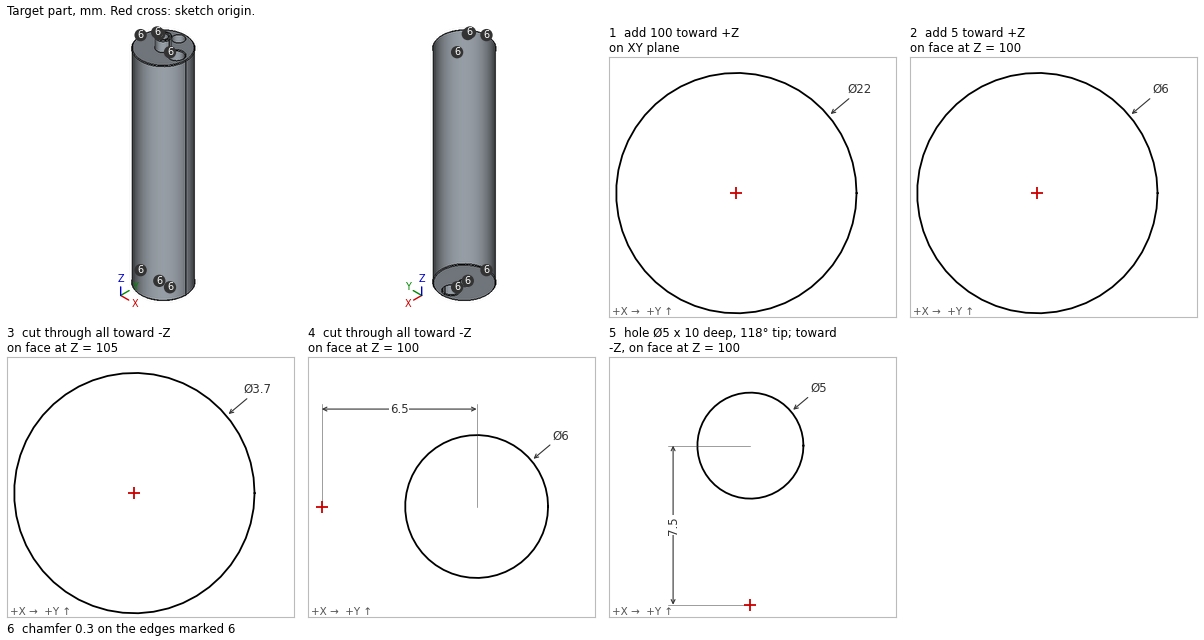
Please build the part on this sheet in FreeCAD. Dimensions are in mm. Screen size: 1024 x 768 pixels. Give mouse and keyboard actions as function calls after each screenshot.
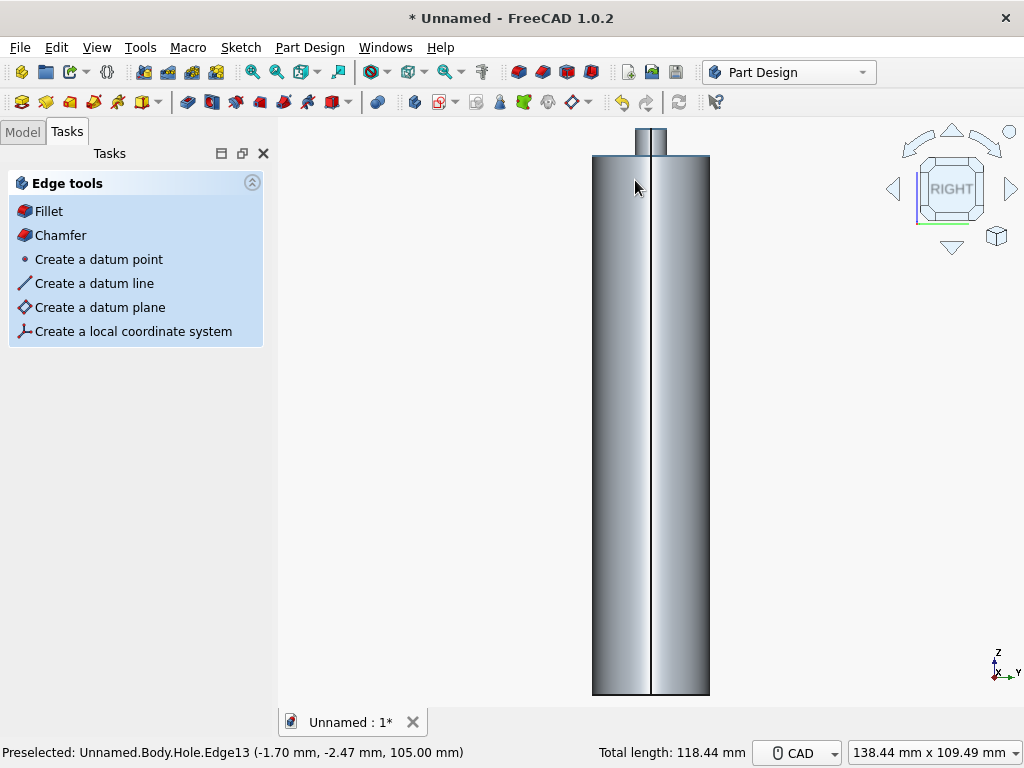
key(5)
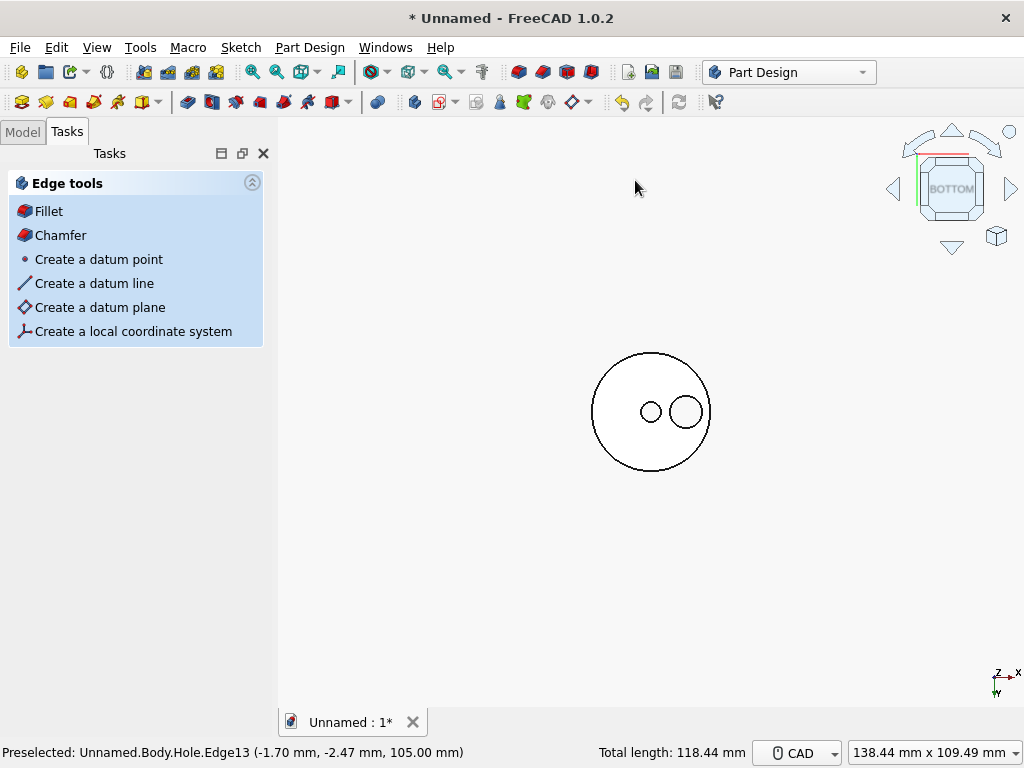
click(254, 72)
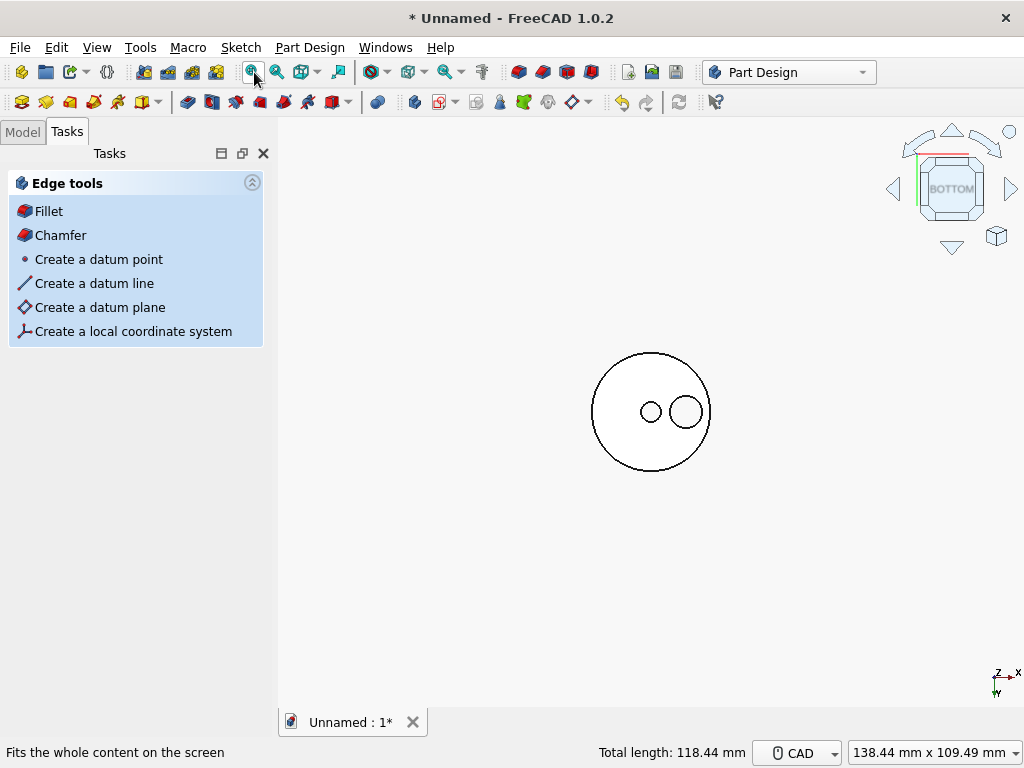
click(651, 377, ctrl)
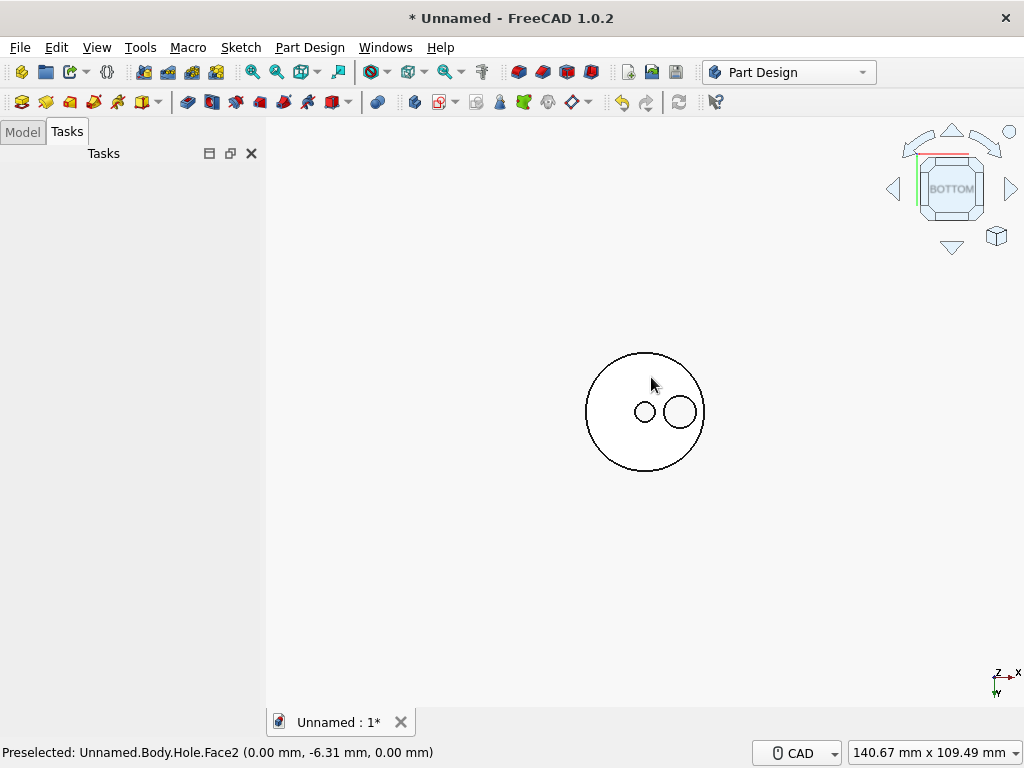
click(544, 72)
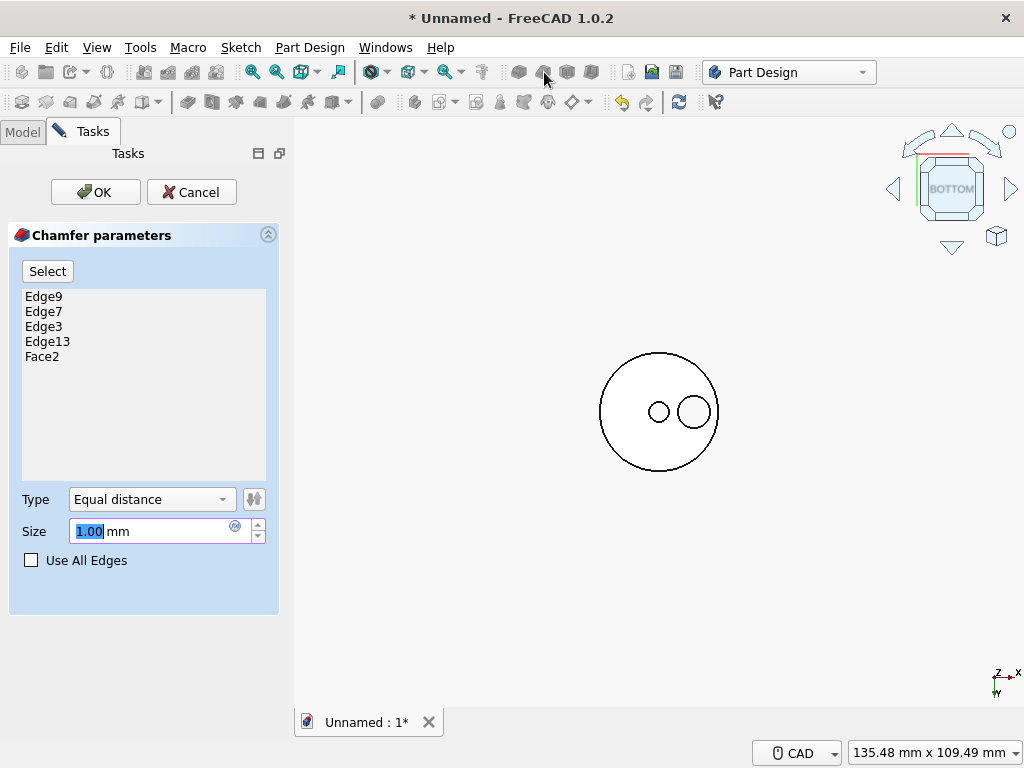
text(0.3)
key(Tab)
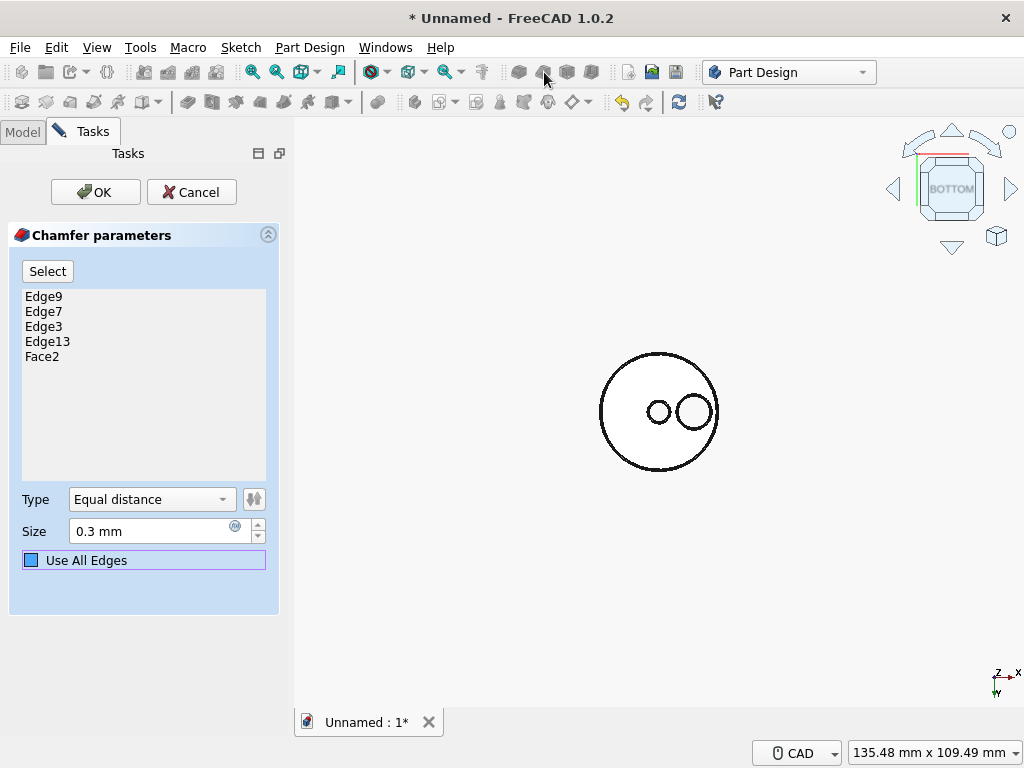
click(96, 192)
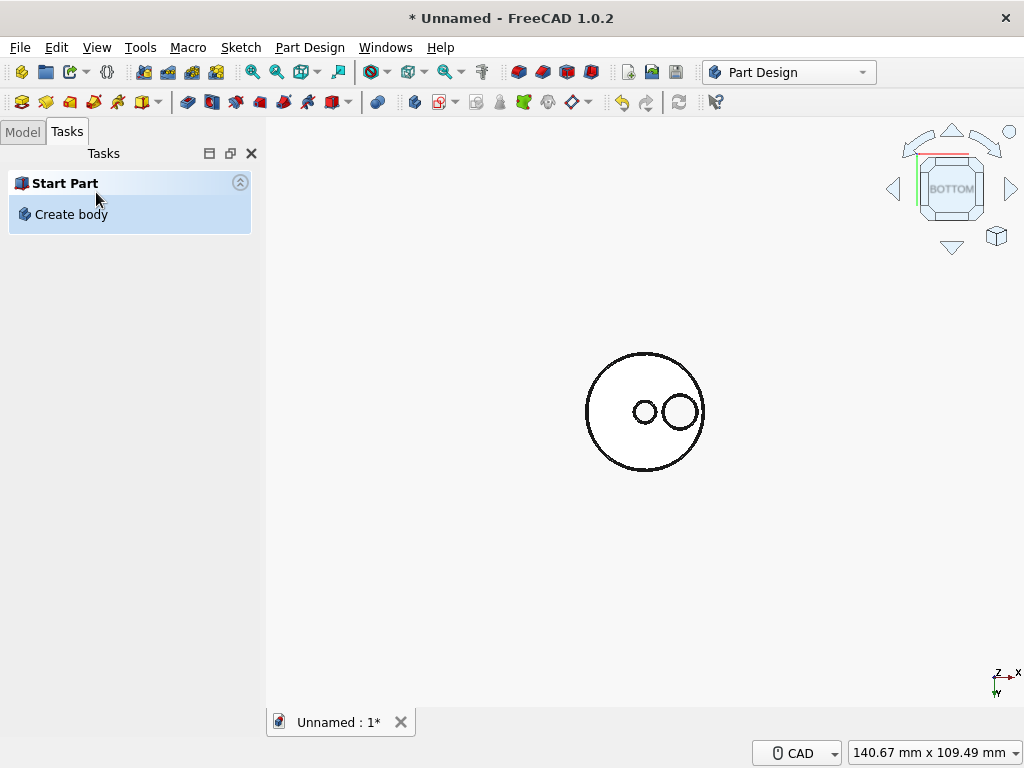
key(0)